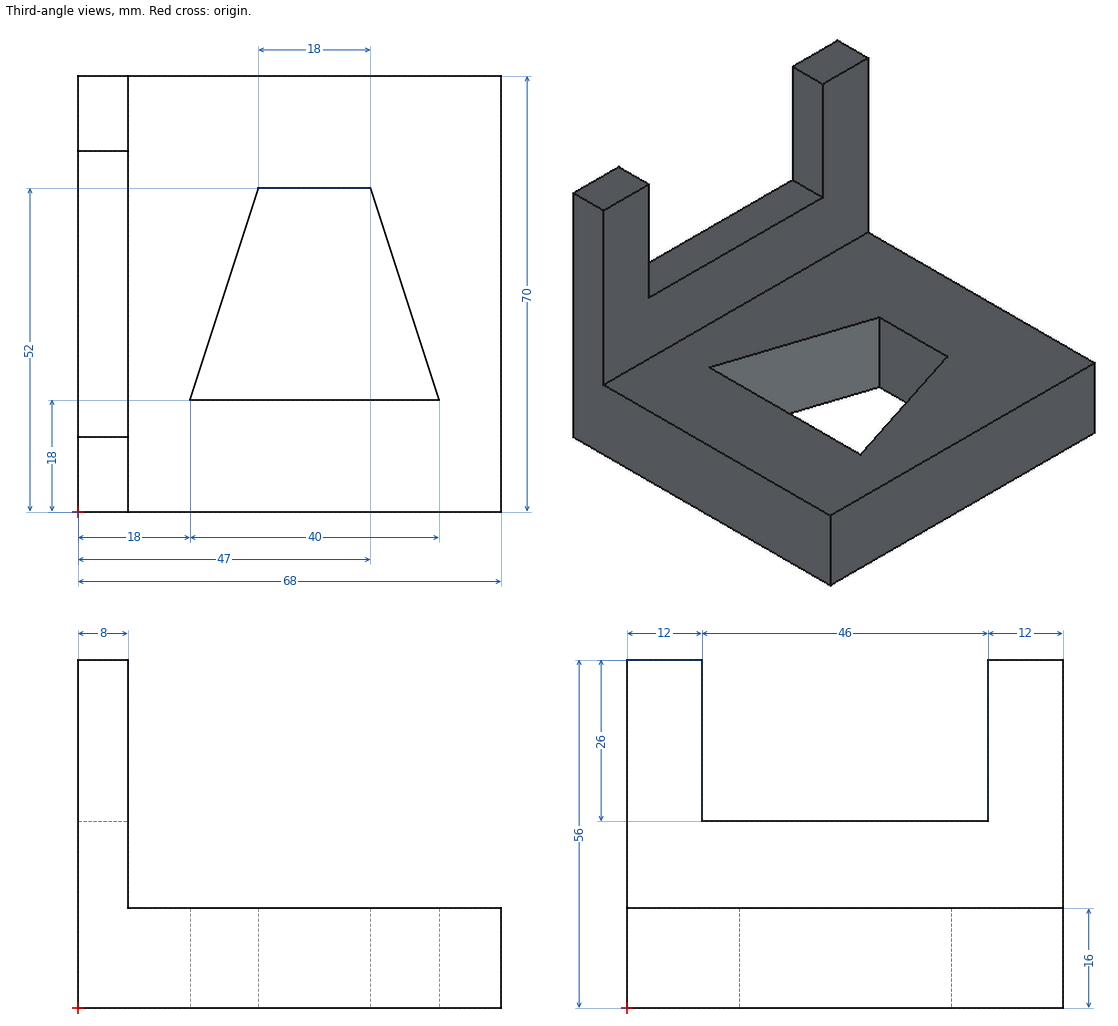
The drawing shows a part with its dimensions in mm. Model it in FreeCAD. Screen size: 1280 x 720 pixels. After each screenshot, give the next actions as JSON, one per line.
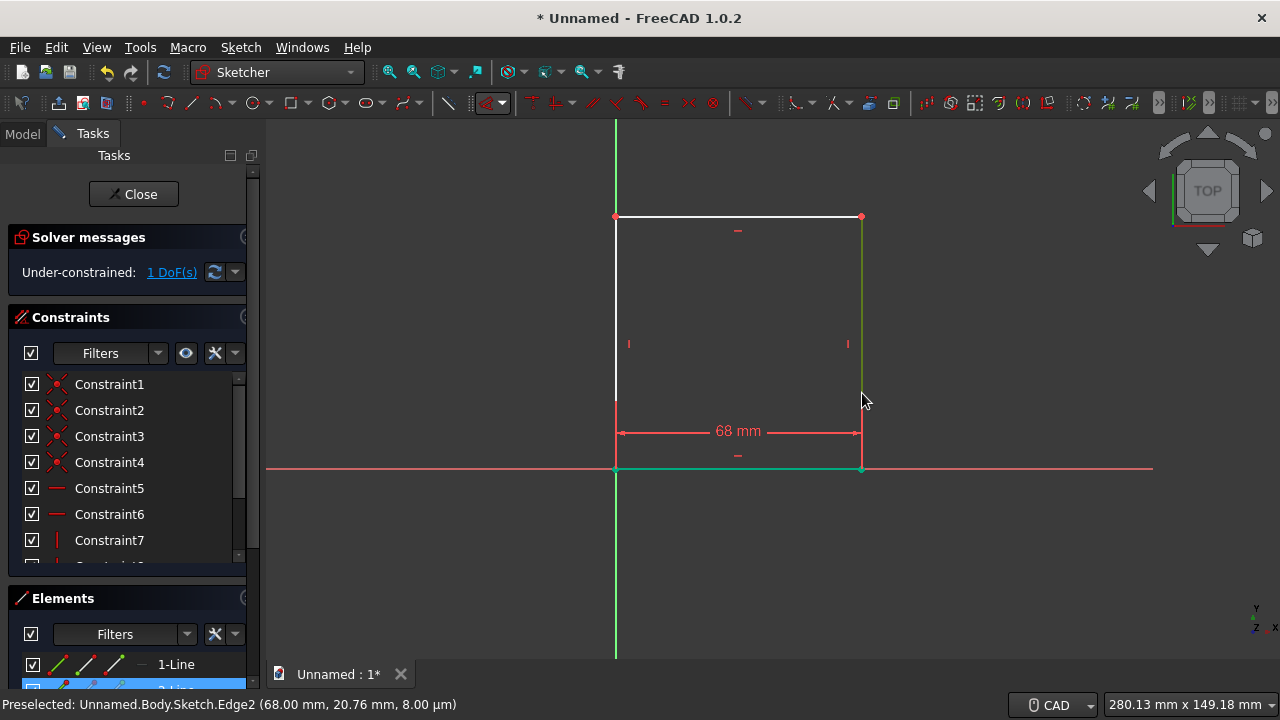
{"action": "key", "text": "i"}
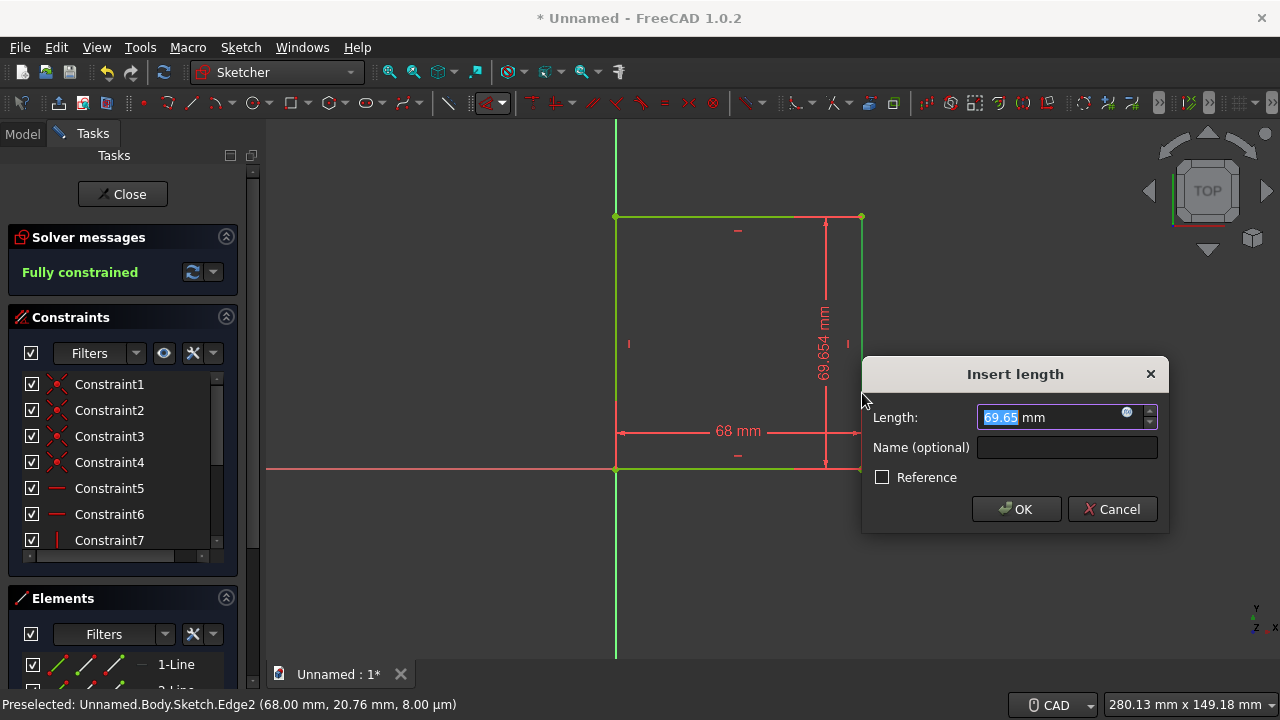
{"action": "type", "text": "70"}
{"action": "key", "text": "Return"}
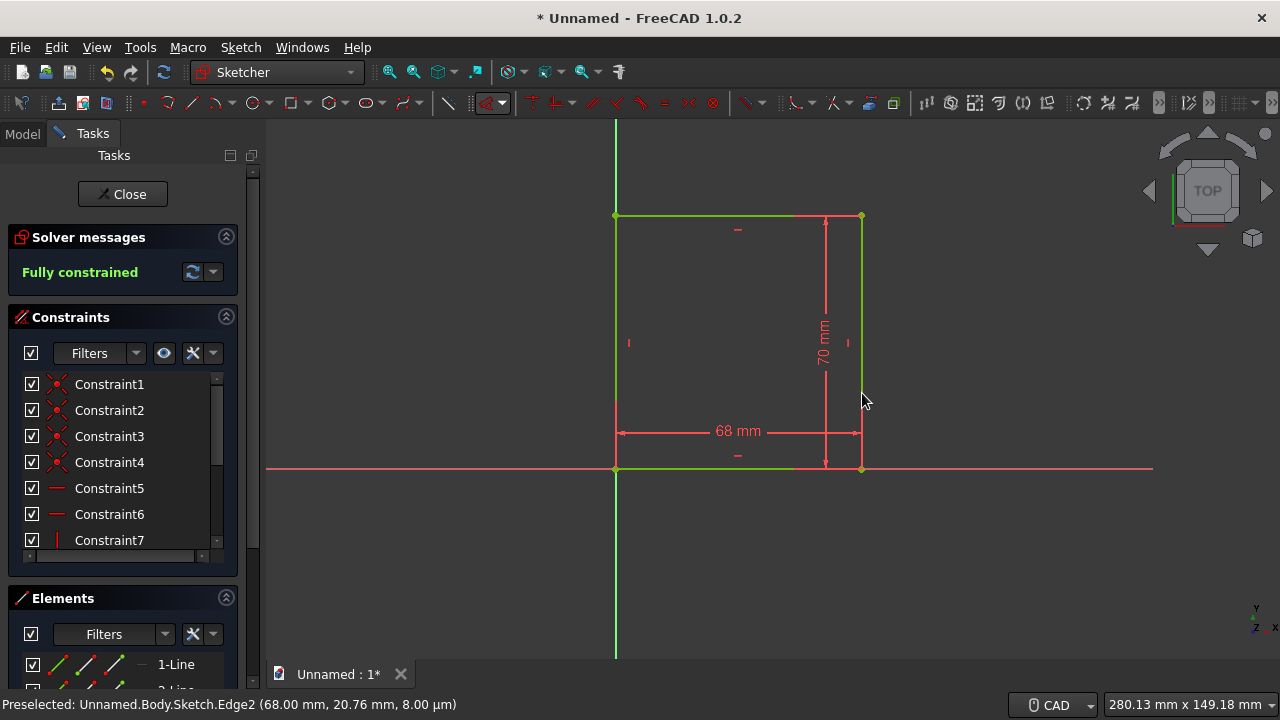
{"action": "left_click", "coordinate": [123, 194]}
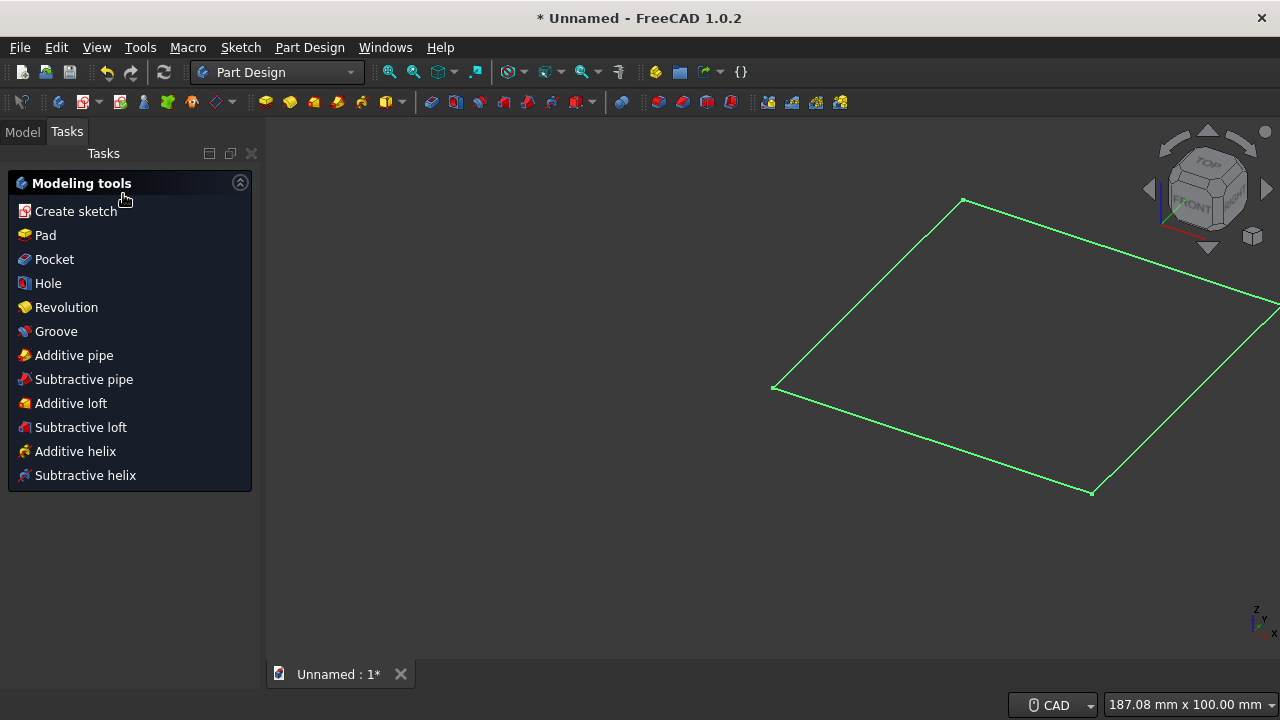
{"action": "left_click", "coordinate": [266, 102]}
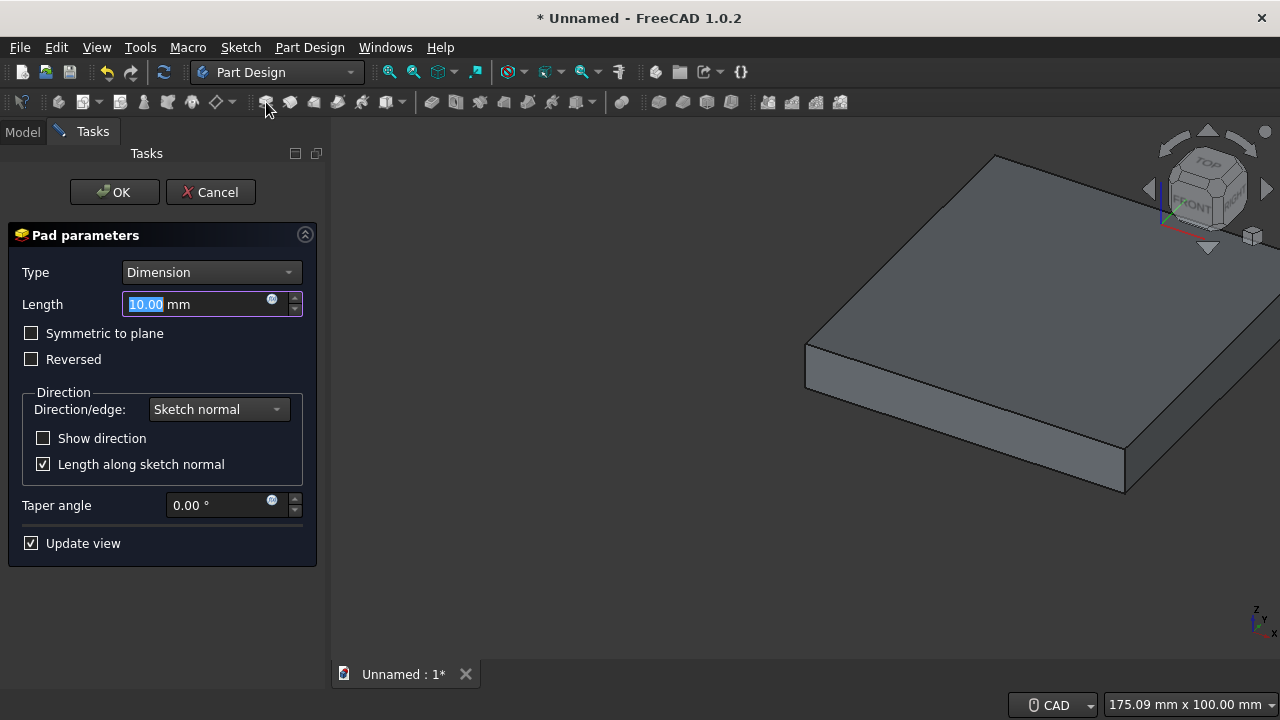
{"action": "type", "text": "16"}
{"action": "key", "text": "Tab"}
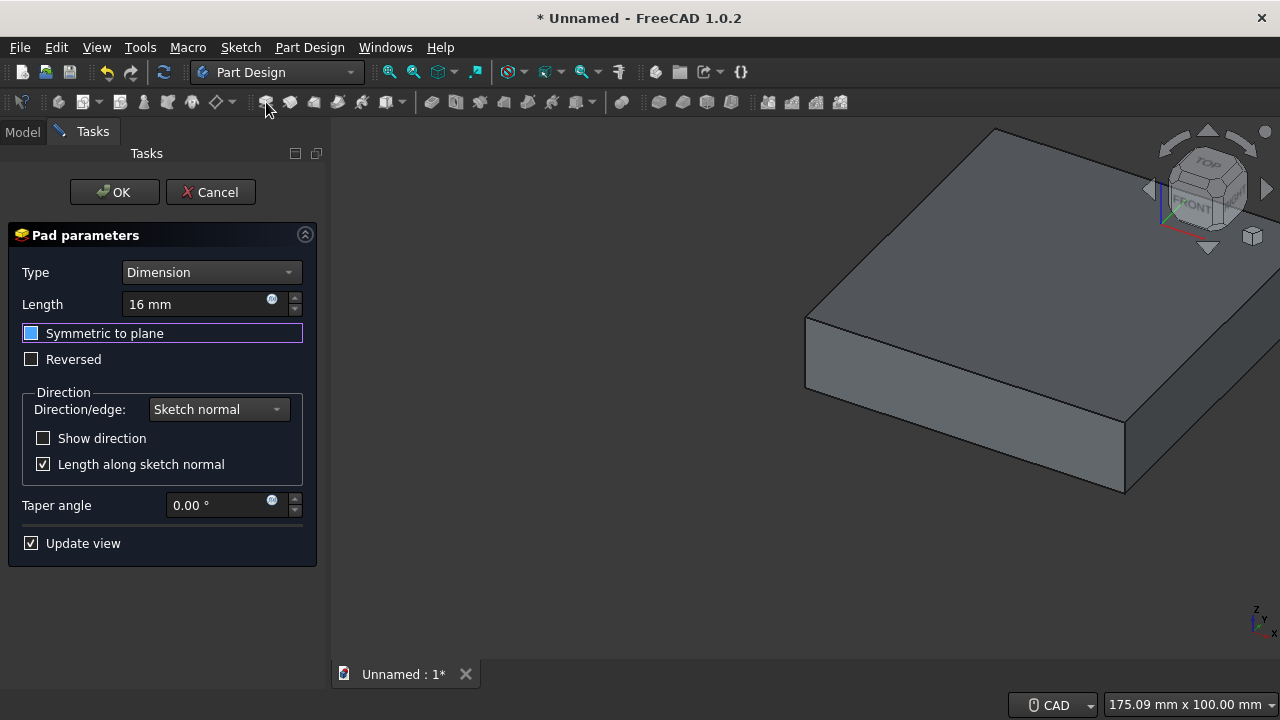
{"action": "left_click", "coordinate": [115, 192]}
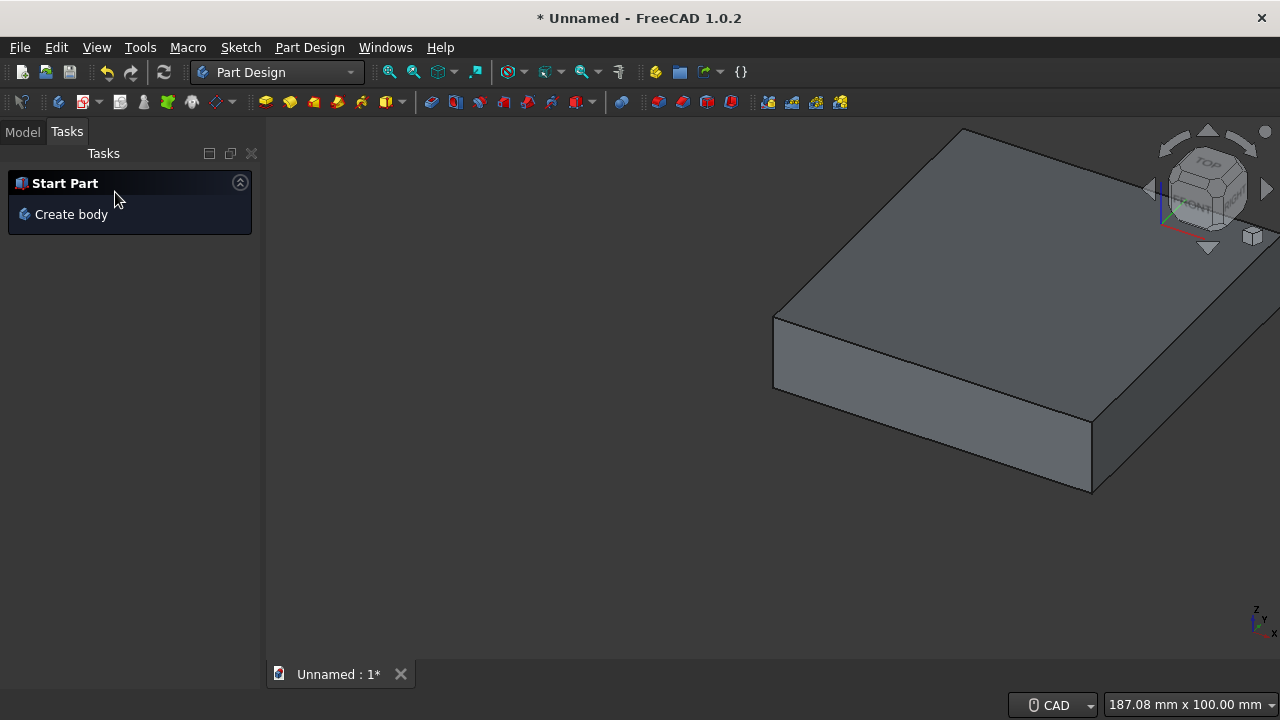
{"action": "key", "text": "v f"}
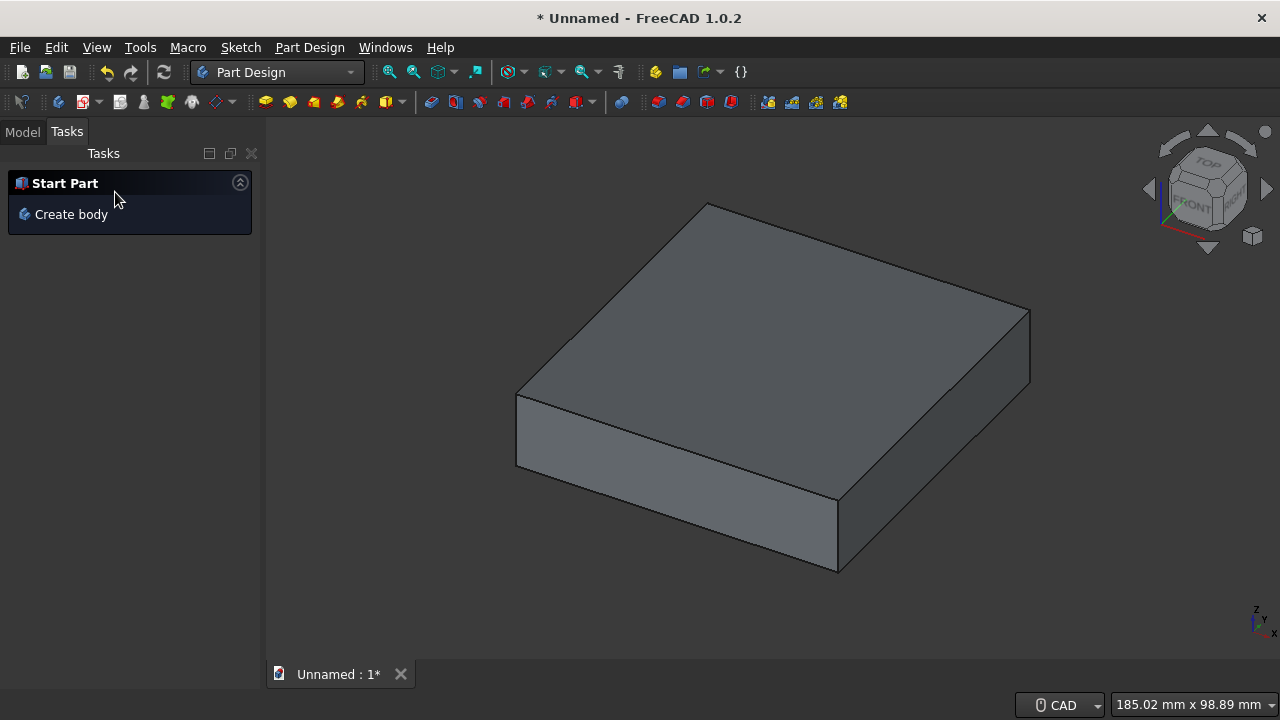
{"action": "left_click", "coordinate": [84, 102]}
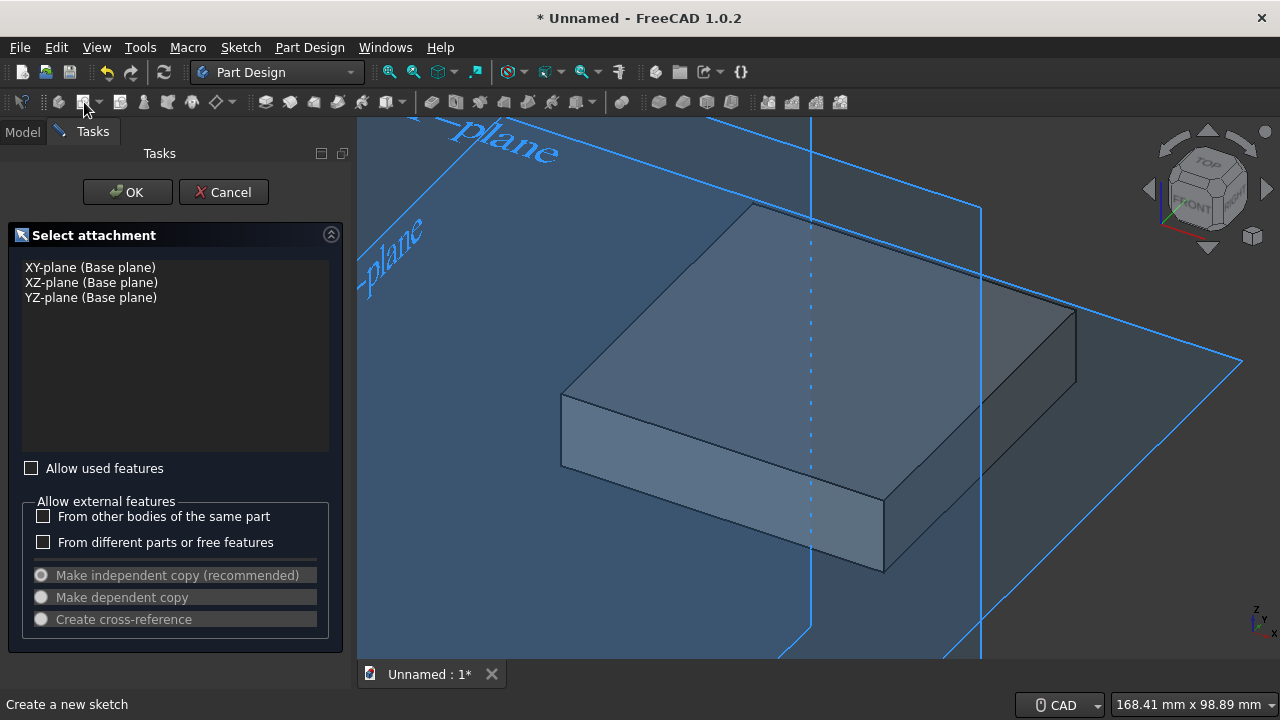
{"action": "left_click", "coordinate": [82, 298]}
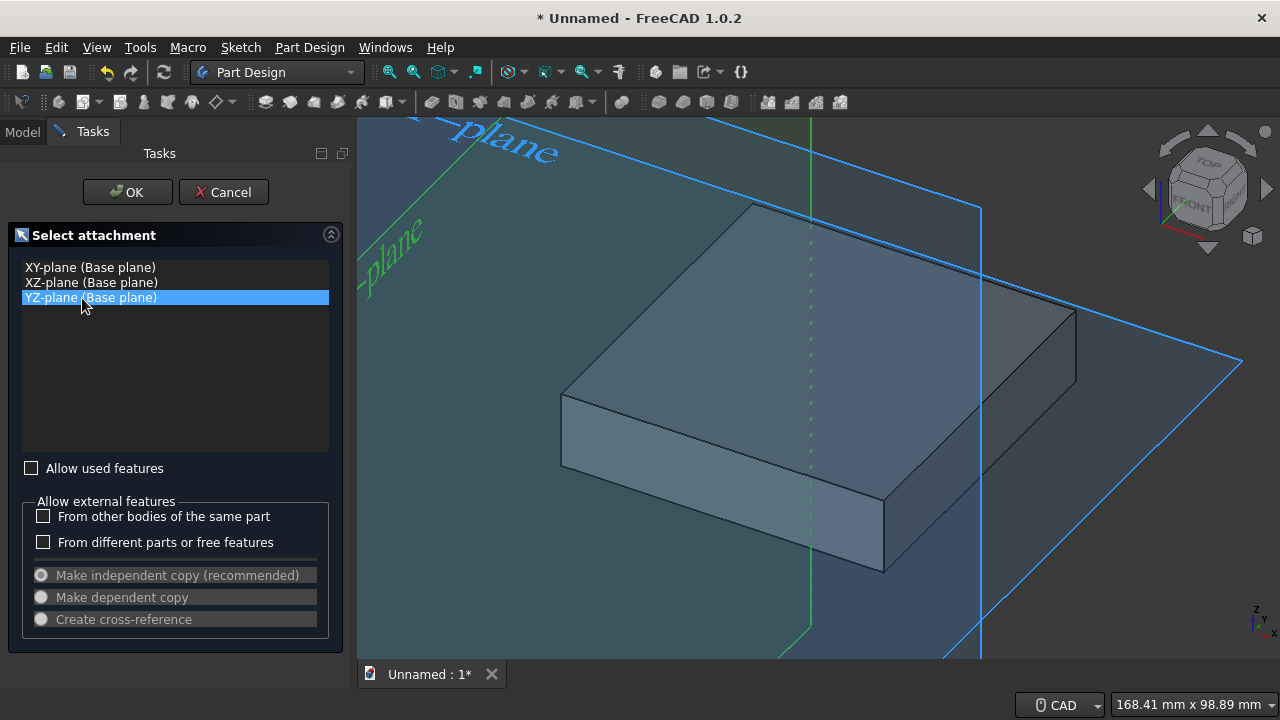
{"action": "left_click", "coordinate": [128, 192]}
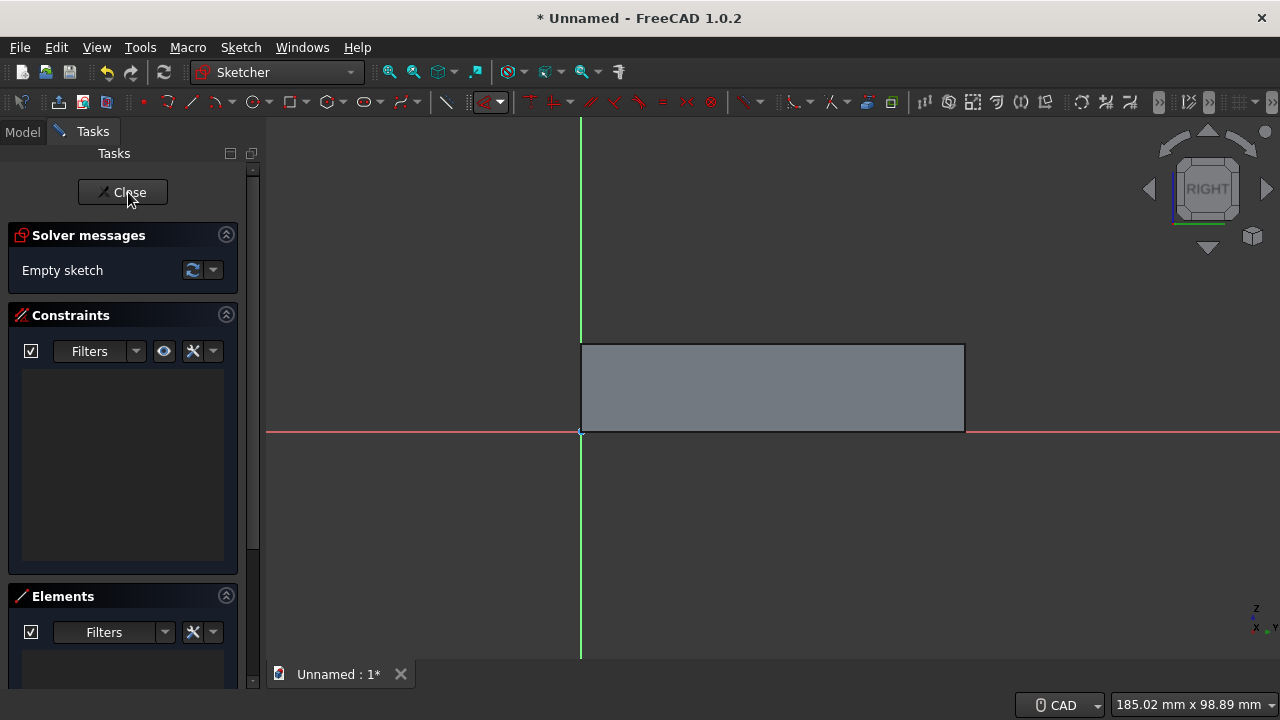
{"action": "key", "text": "q s"}